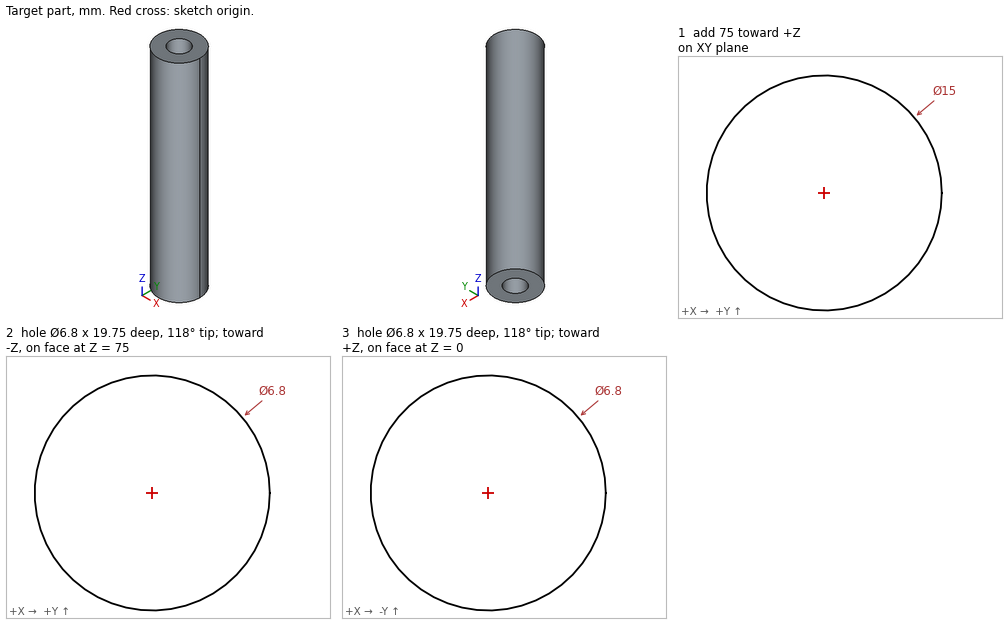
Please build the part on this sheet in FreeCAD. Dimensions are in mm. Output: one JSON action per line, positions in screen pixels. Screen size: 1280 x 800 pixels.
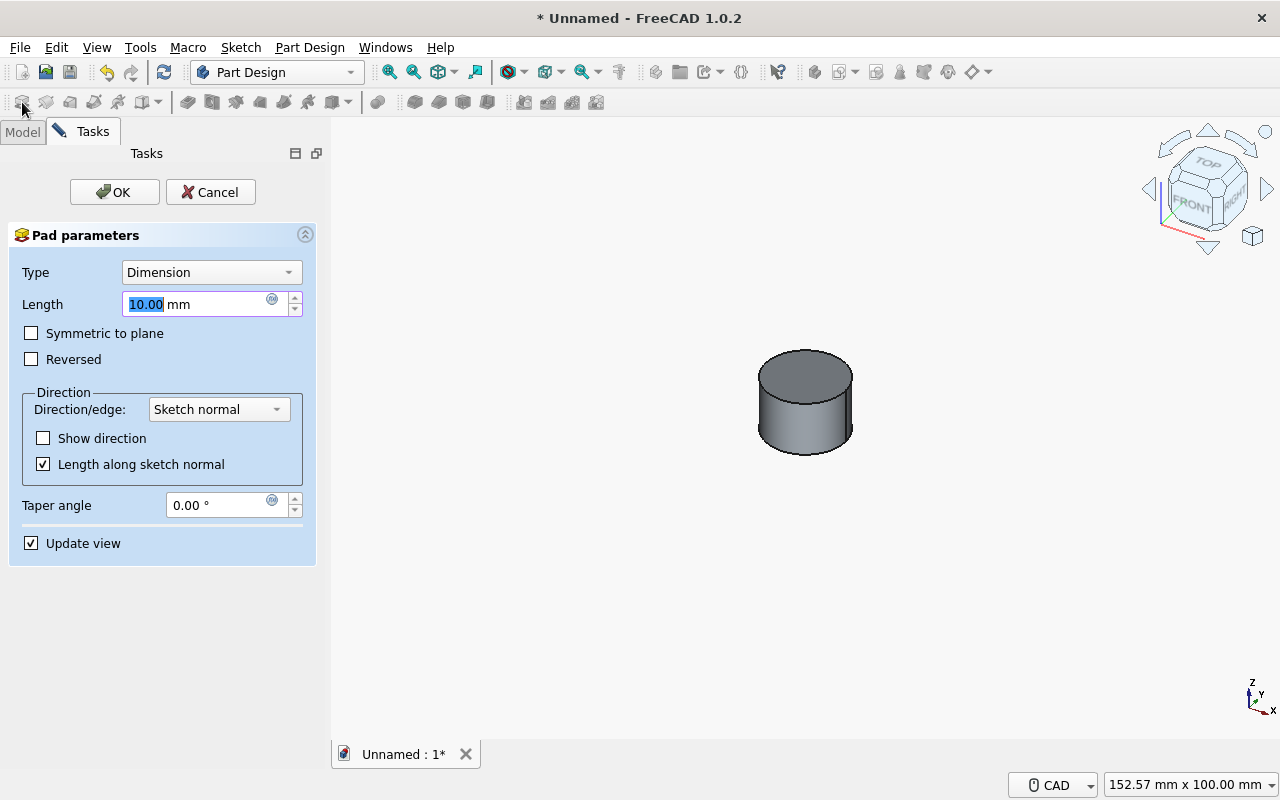
{"action": "type", "text": "75"}
{"action": "key", "text": "Tab"}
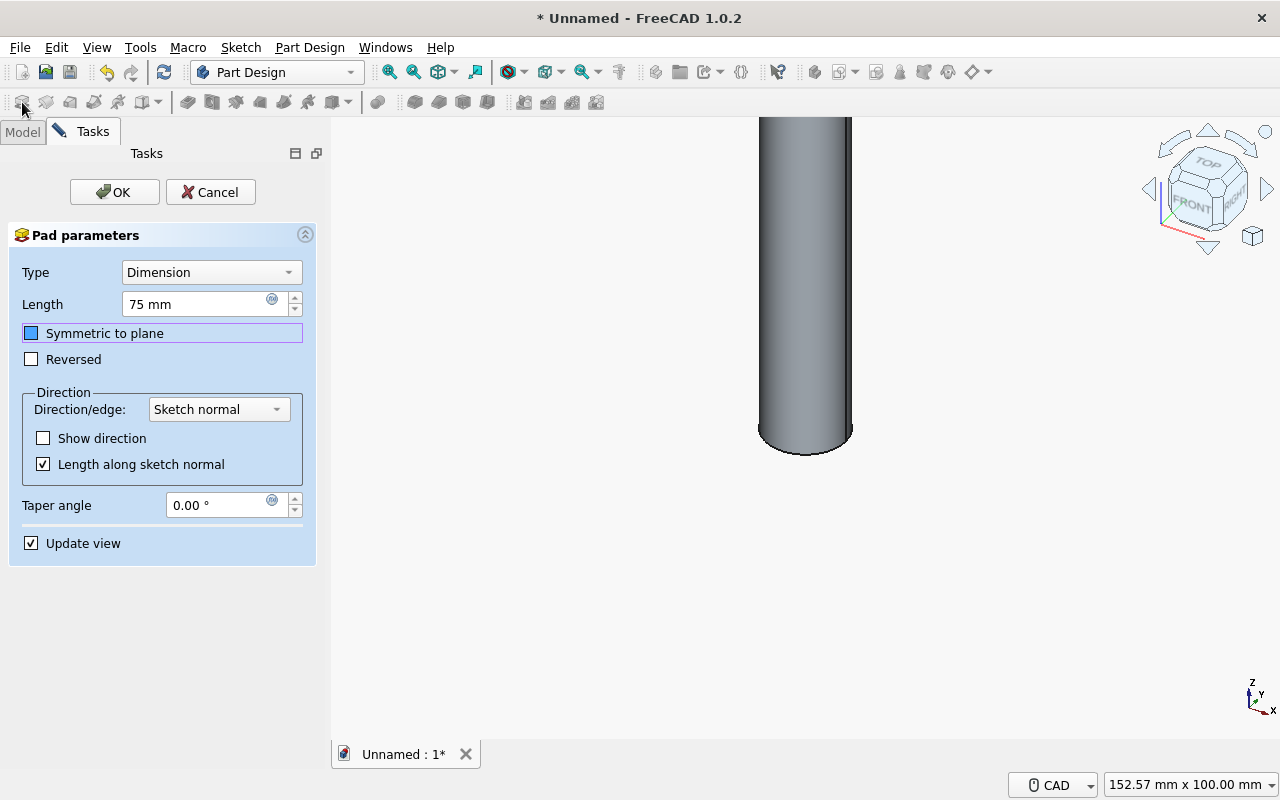
{"action": "left_click", "coordinate": [115, 192]}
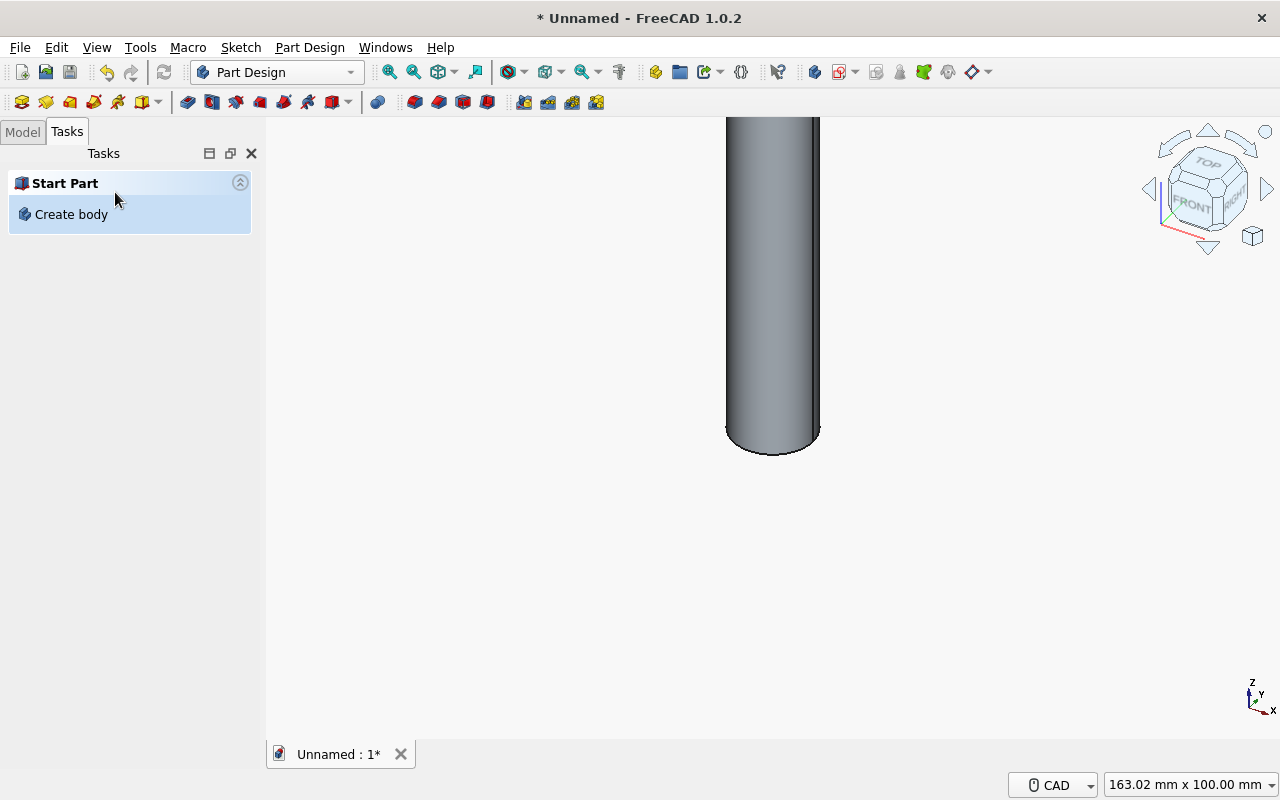
{"action": "left_click", "coordinate": [390, 72]}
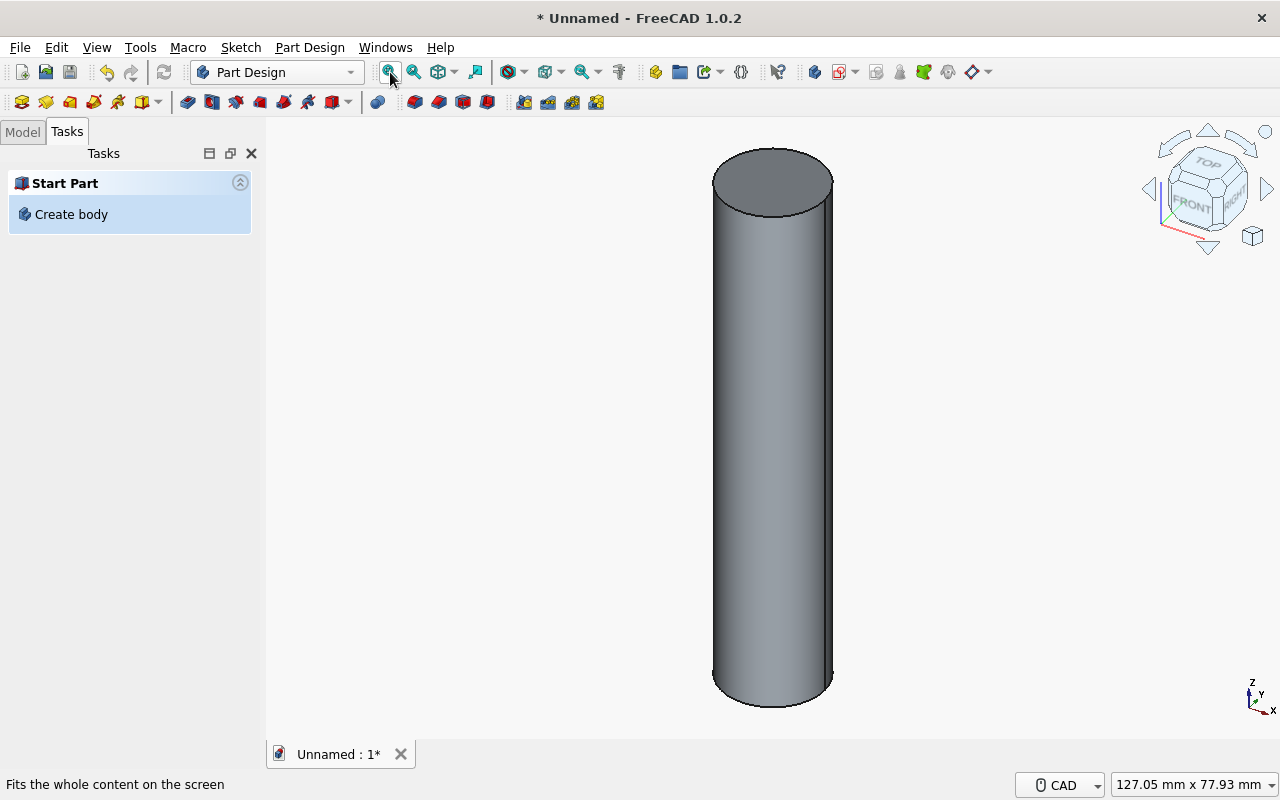
{"action": "left_click", "coordinate": [773, 182]}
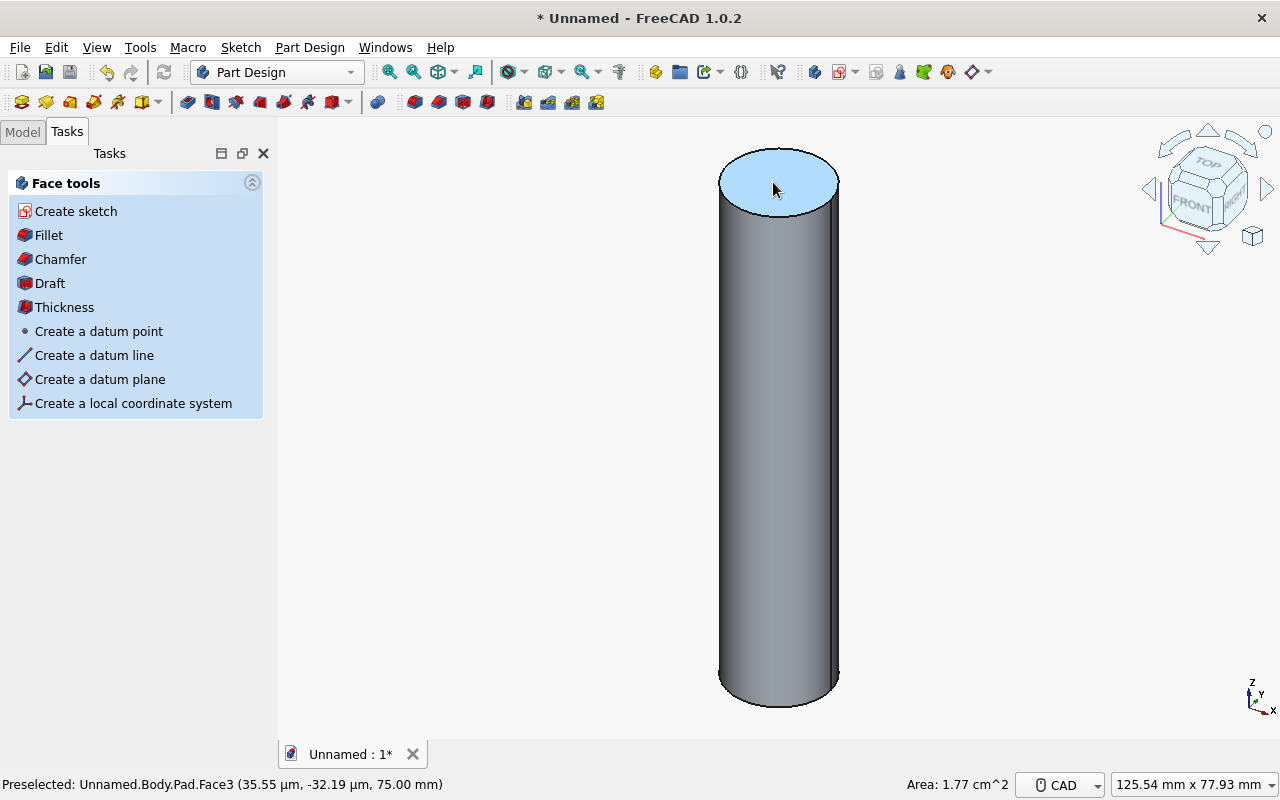
{"action": "left_click", "coordinate": [840, 72]}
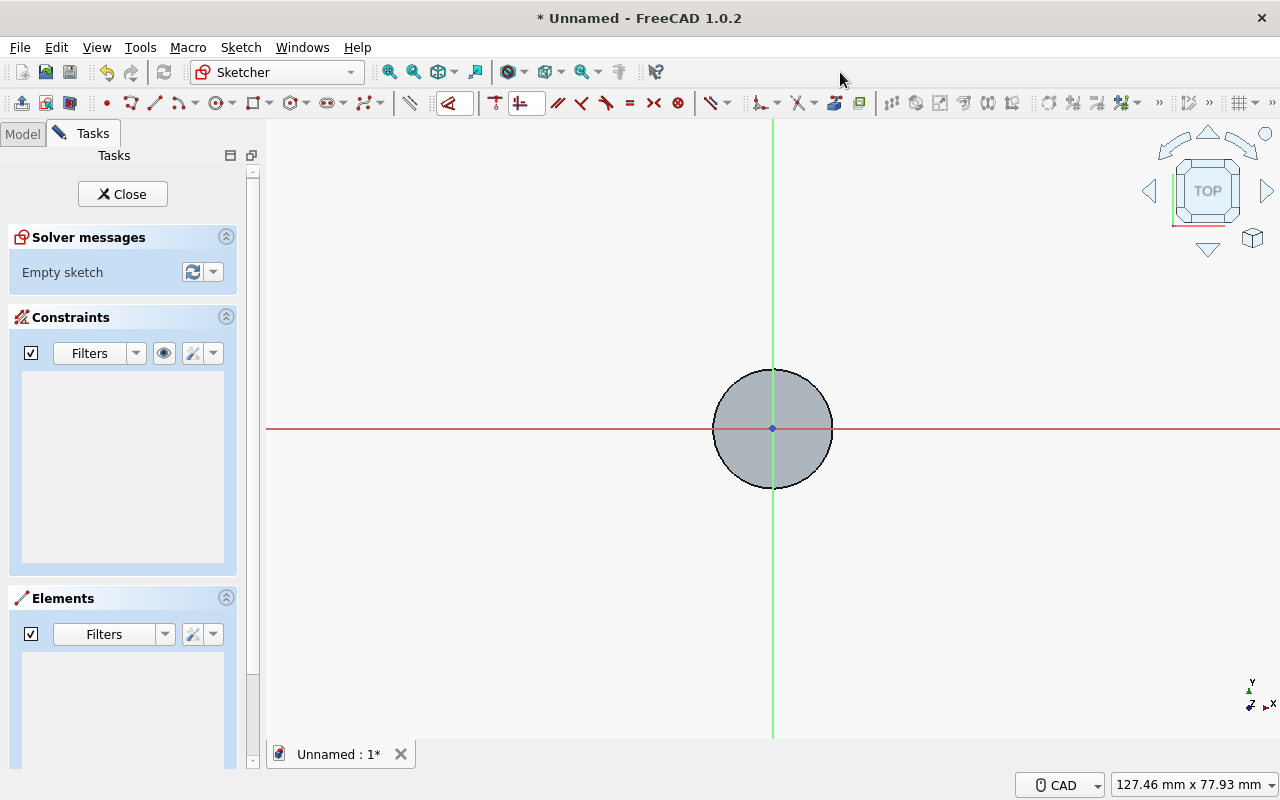
{"action": "scroll", "coordinate": [784, 429], "scroll_direction": "up", "scroll_amount": 10}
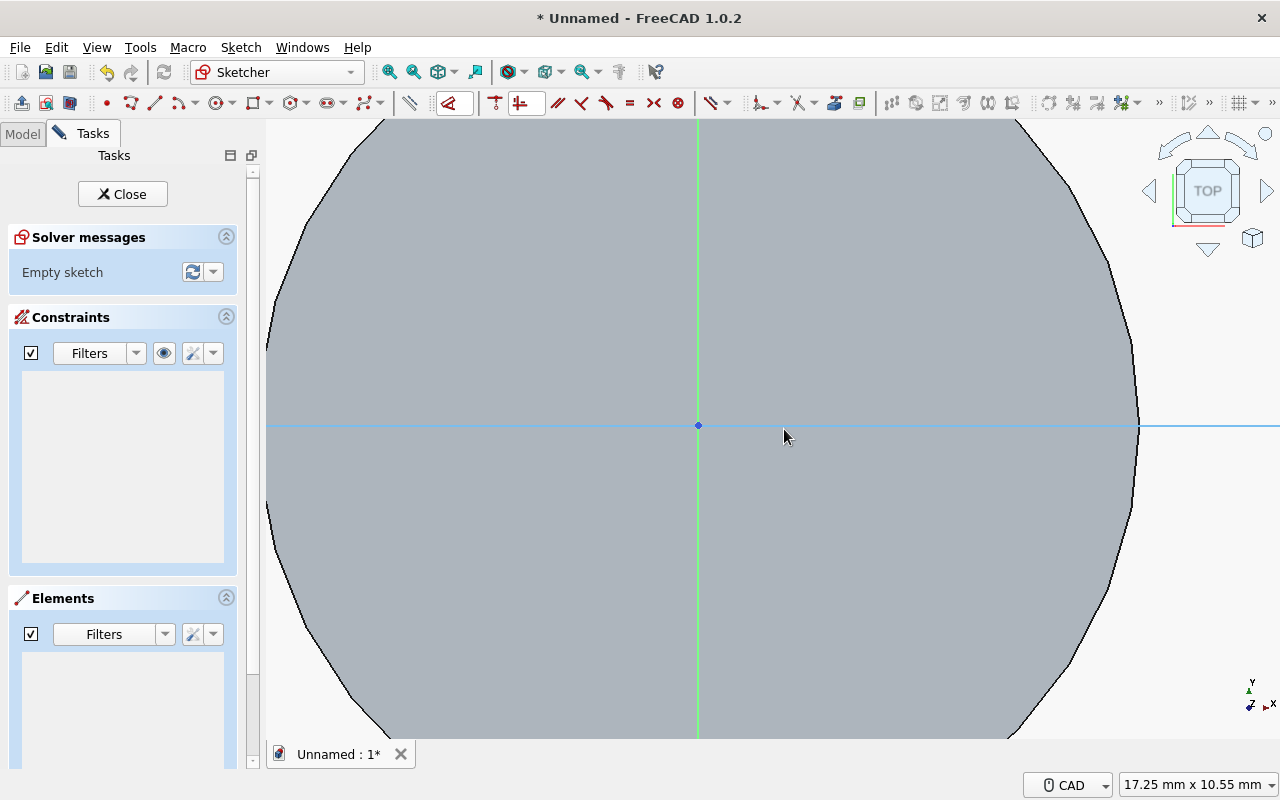
{"action": "key", "text": "g c"}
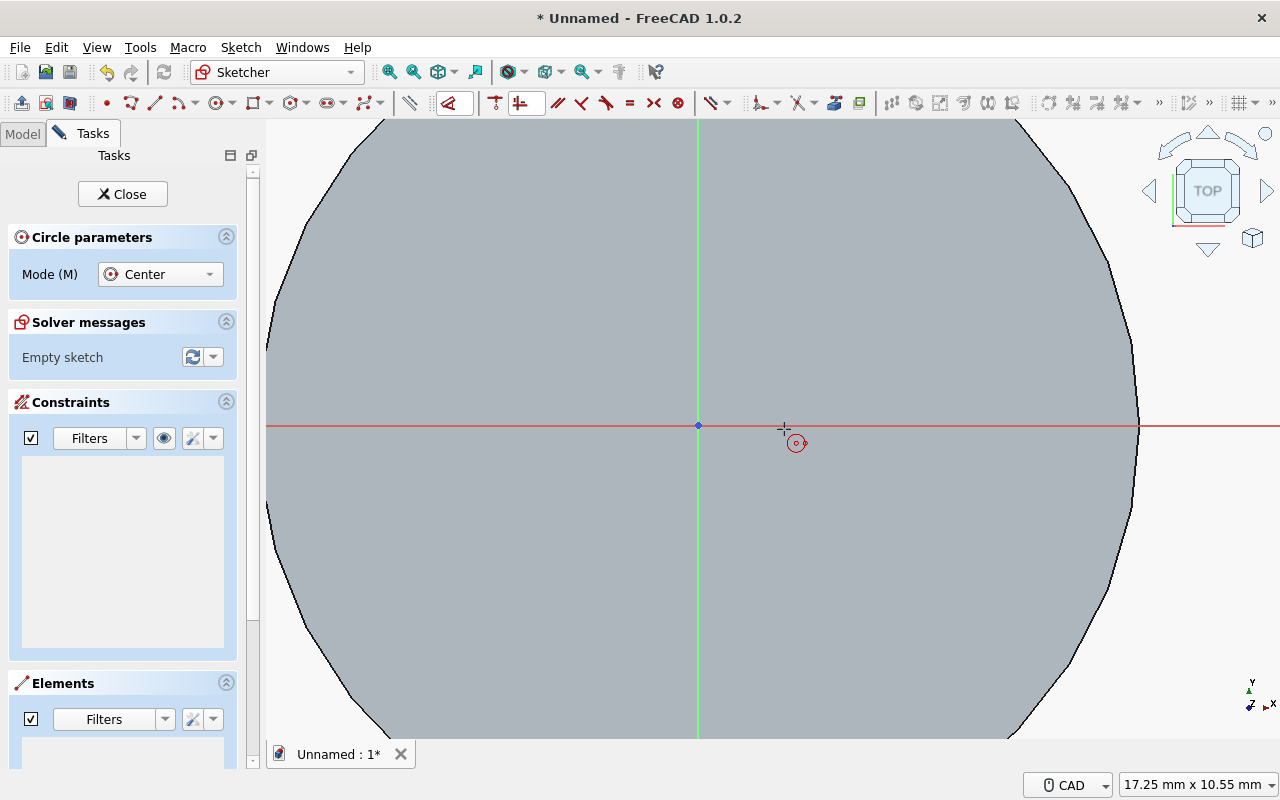
{"action": "left_click", "coordinate": [698, 426]}
{"action": "mouse_move", "coordinate": [840, 284]}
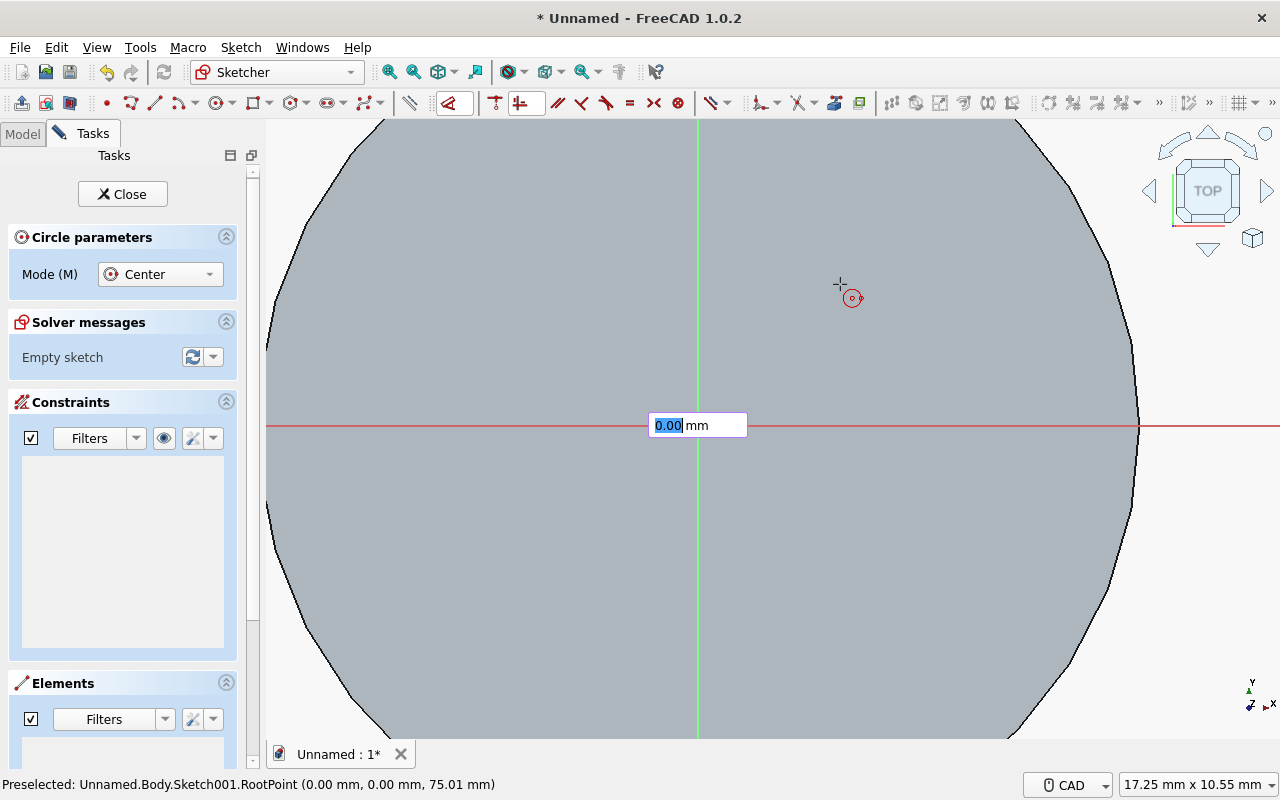
{"action": "type", "text": "6.8"}
{"action": "key", "text": "Return"}
{"action": "key", "text": "Escape"}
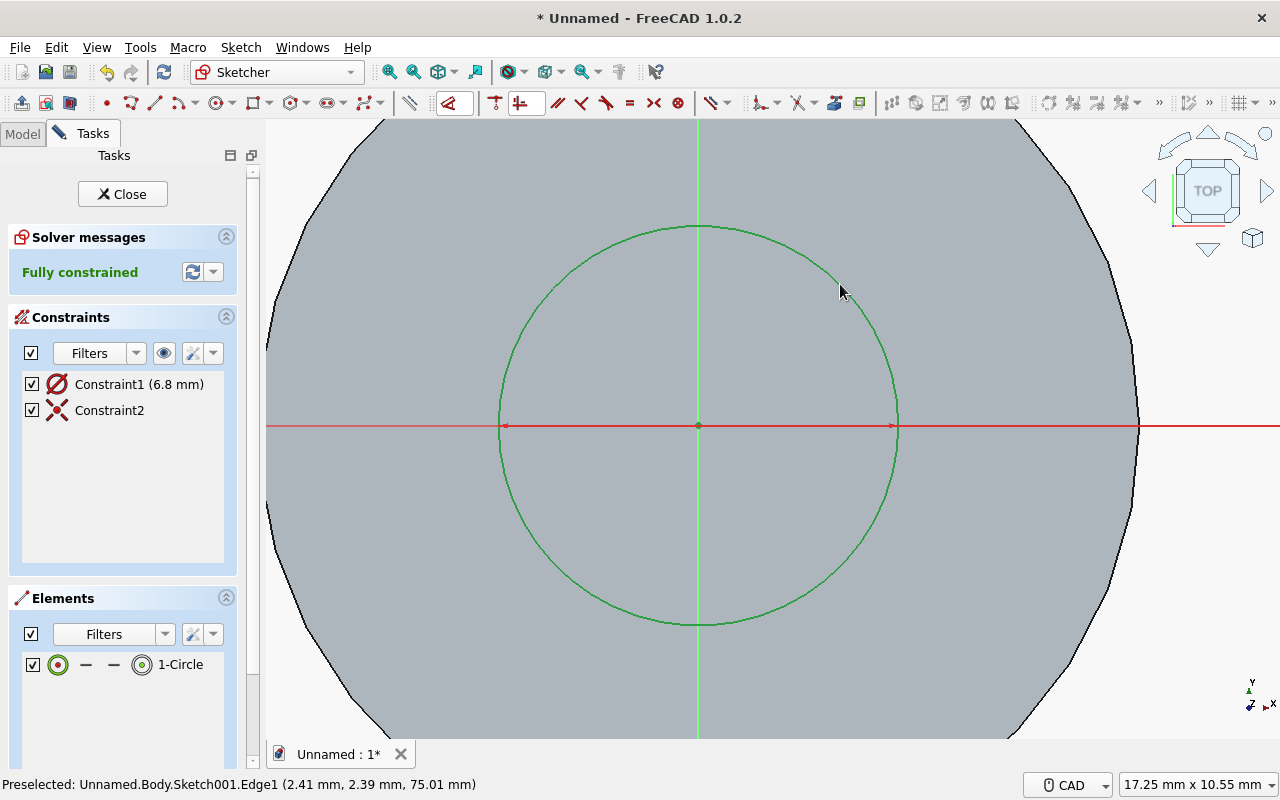
{"action": "left_click", "coordinate": [123, 194]}